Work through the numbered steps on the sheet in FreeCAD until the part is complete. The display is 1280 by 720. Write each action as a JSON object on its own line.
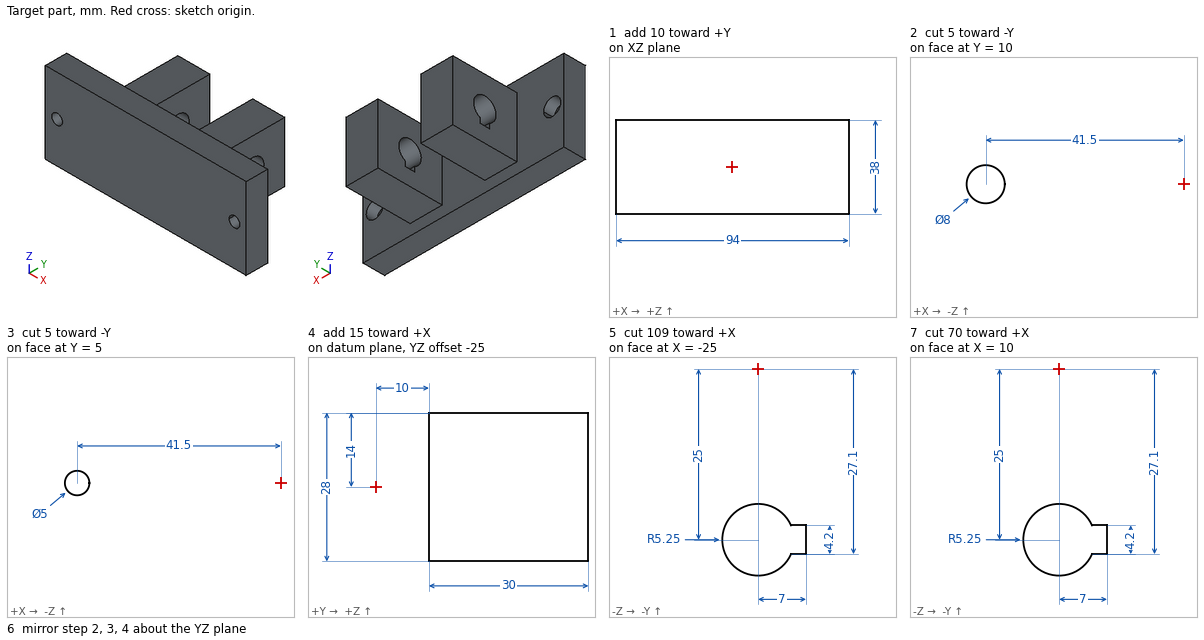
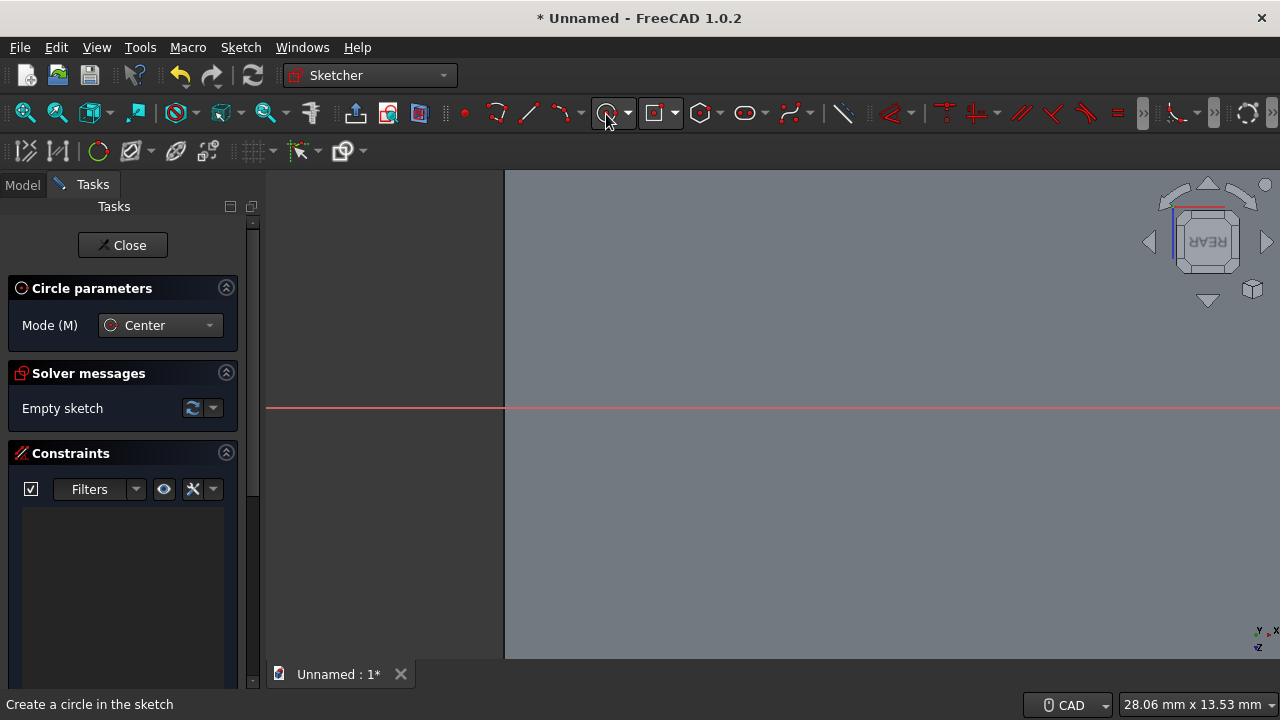
{"action": "left_click", "coordinate": [703, 408]}
{"action": "left_click", "coordinate": [805, 306]}
{"action": "key", "text": "Escape"}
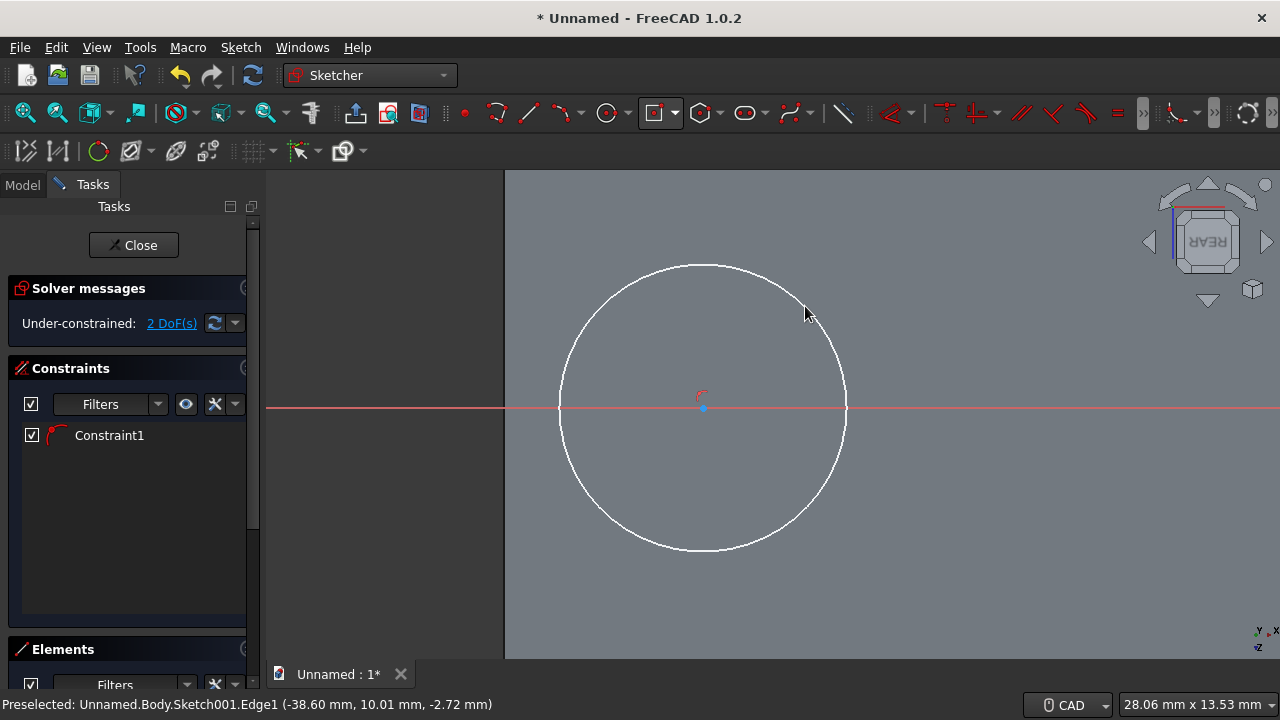
{"action": "left_click", "coordinate": [890, 114]}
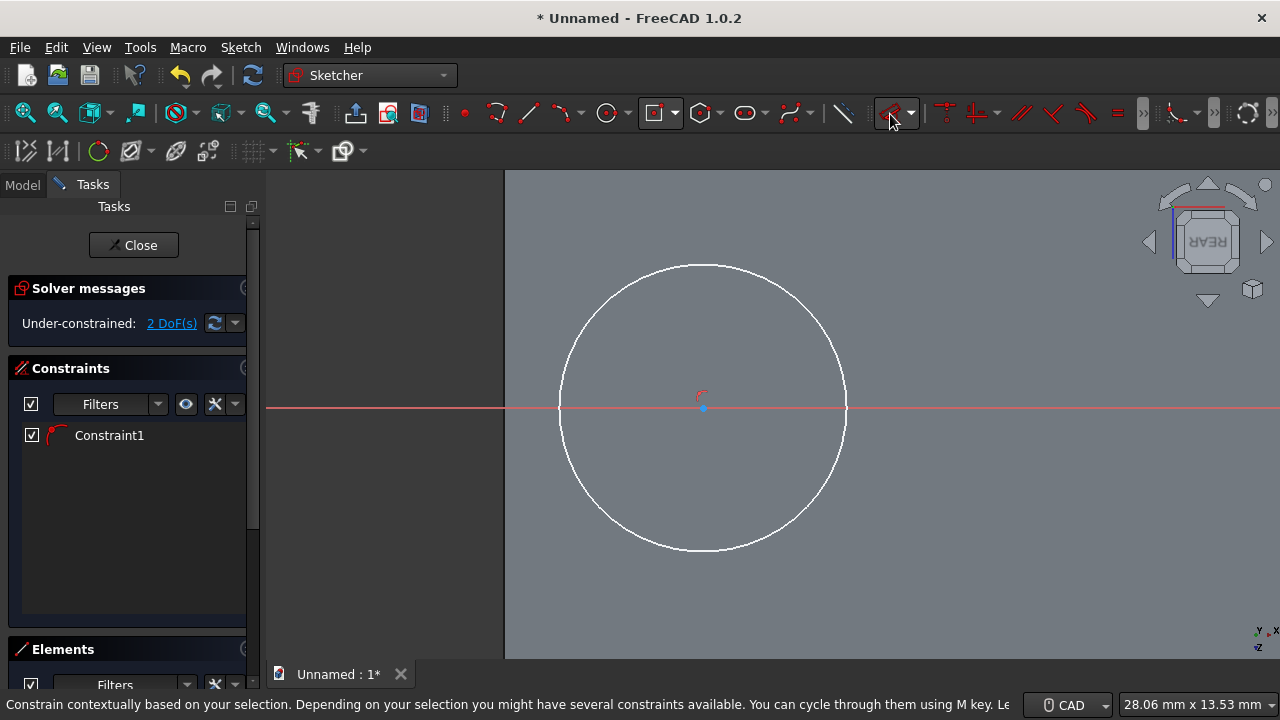
{"action": "left_click", "coordinate": [804, 306]}
{"action": "left_click", "coordinate": [827, 283]}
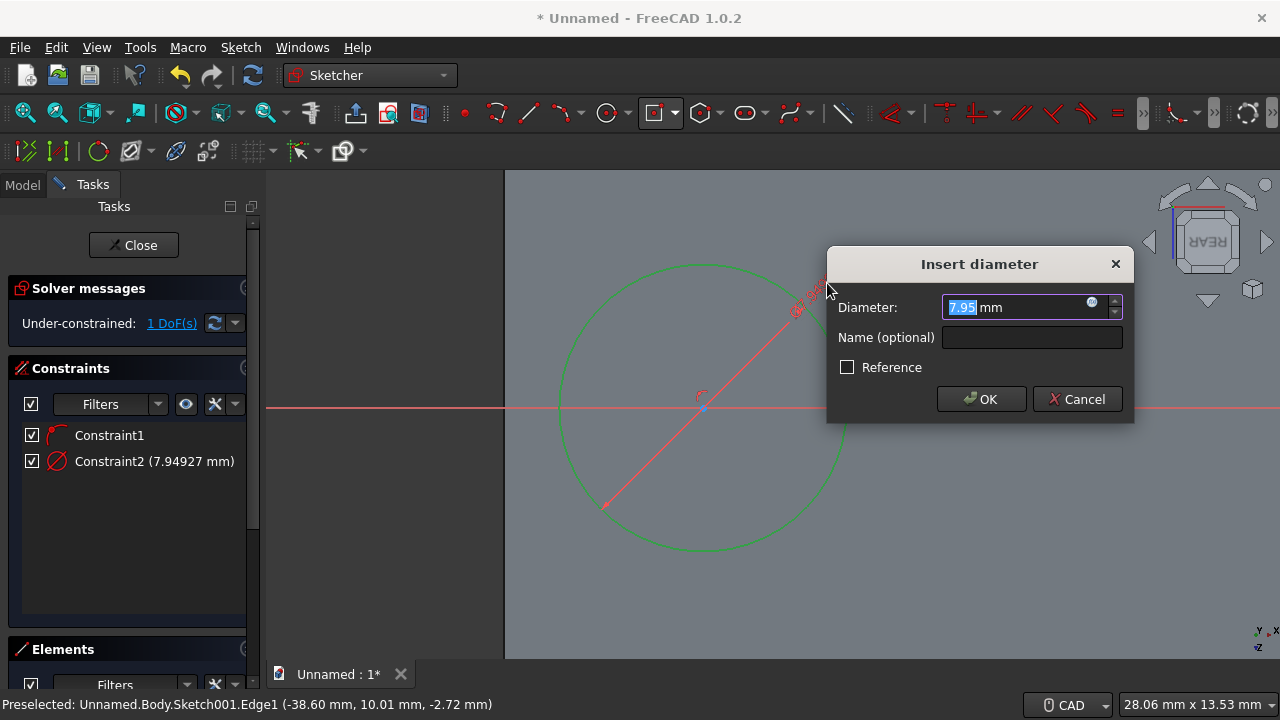
{"action": "type", "text": "8"}
{"action": "key", "text": "Return"}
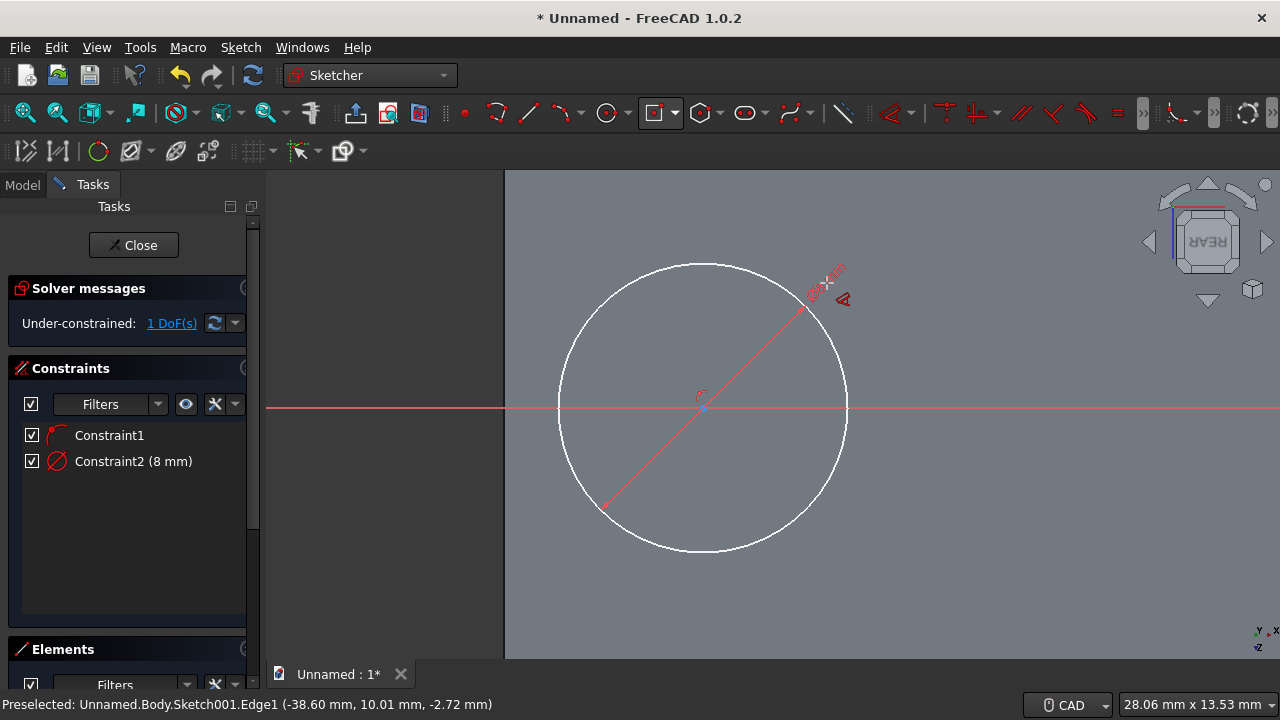
{"action": "left_click", "coordinate": [703, 408]}
{"action": "left_click", "coordinate": [909, 442]}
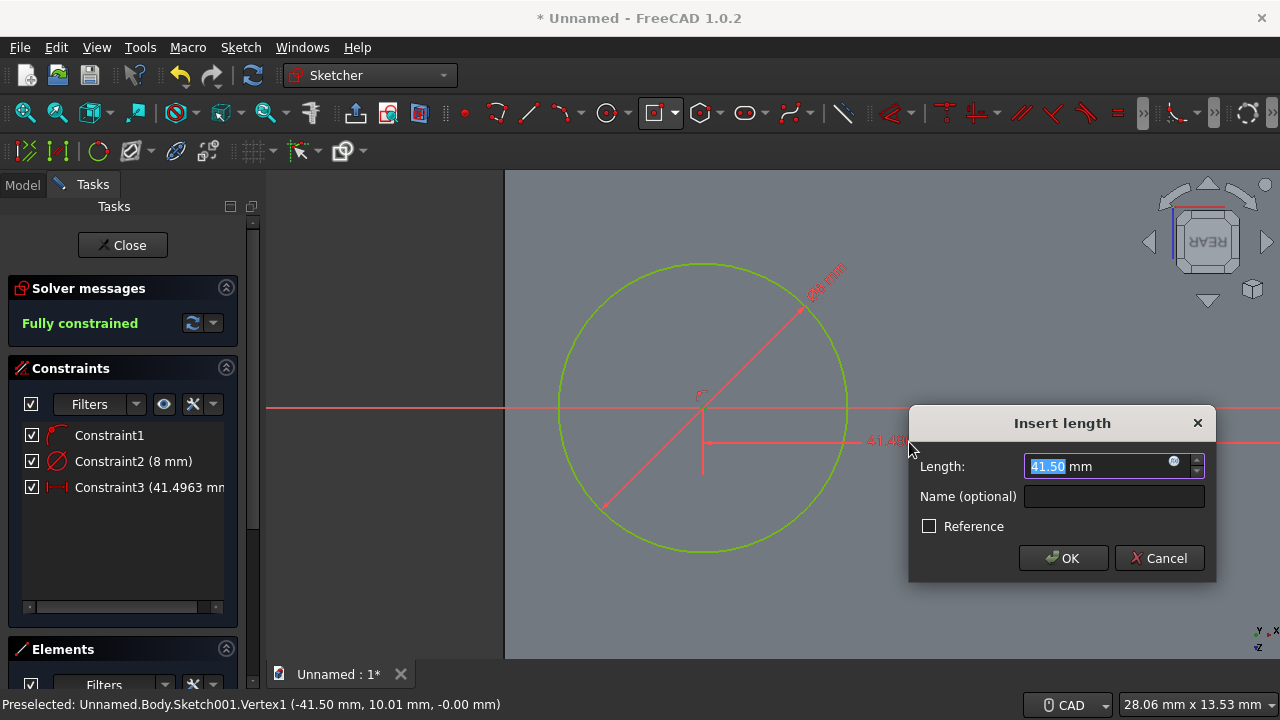
{"action": "type", "text": "41.5"}
{"action": "key", "text": "Return"}
{"action": "key", "text": "Escape"}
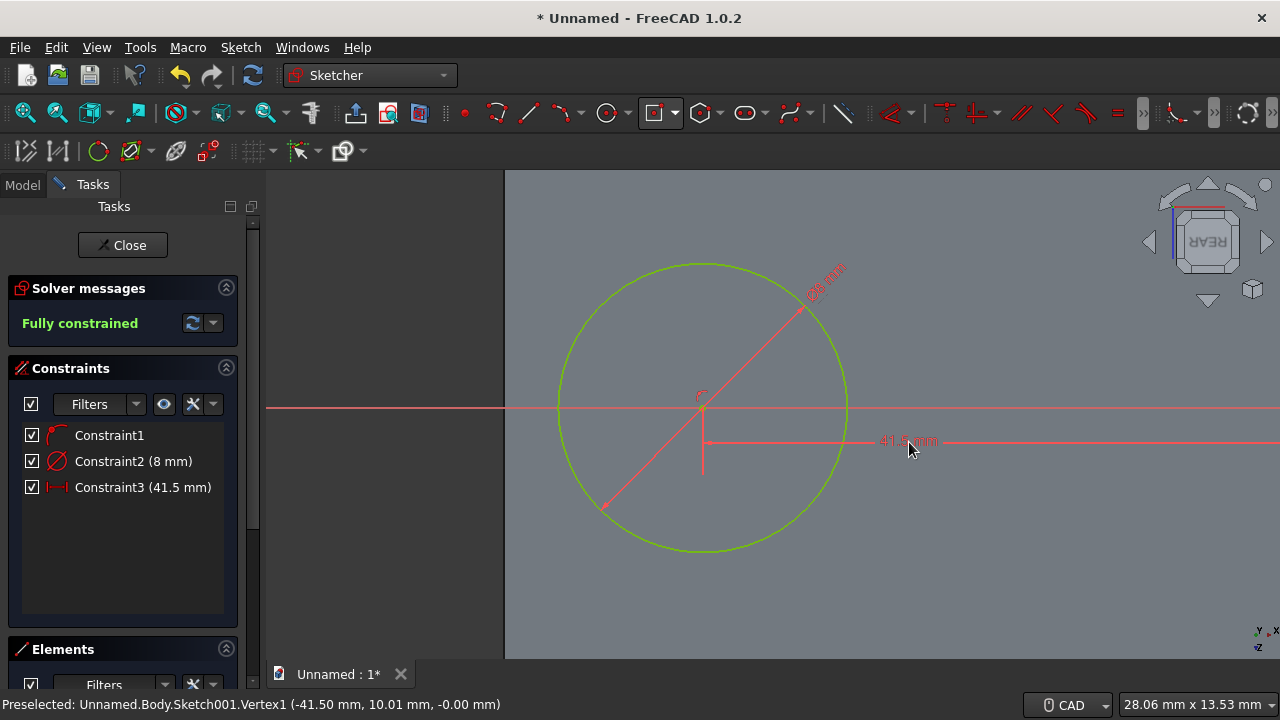
{"action": "left_click", "coordinate": [123, 245]}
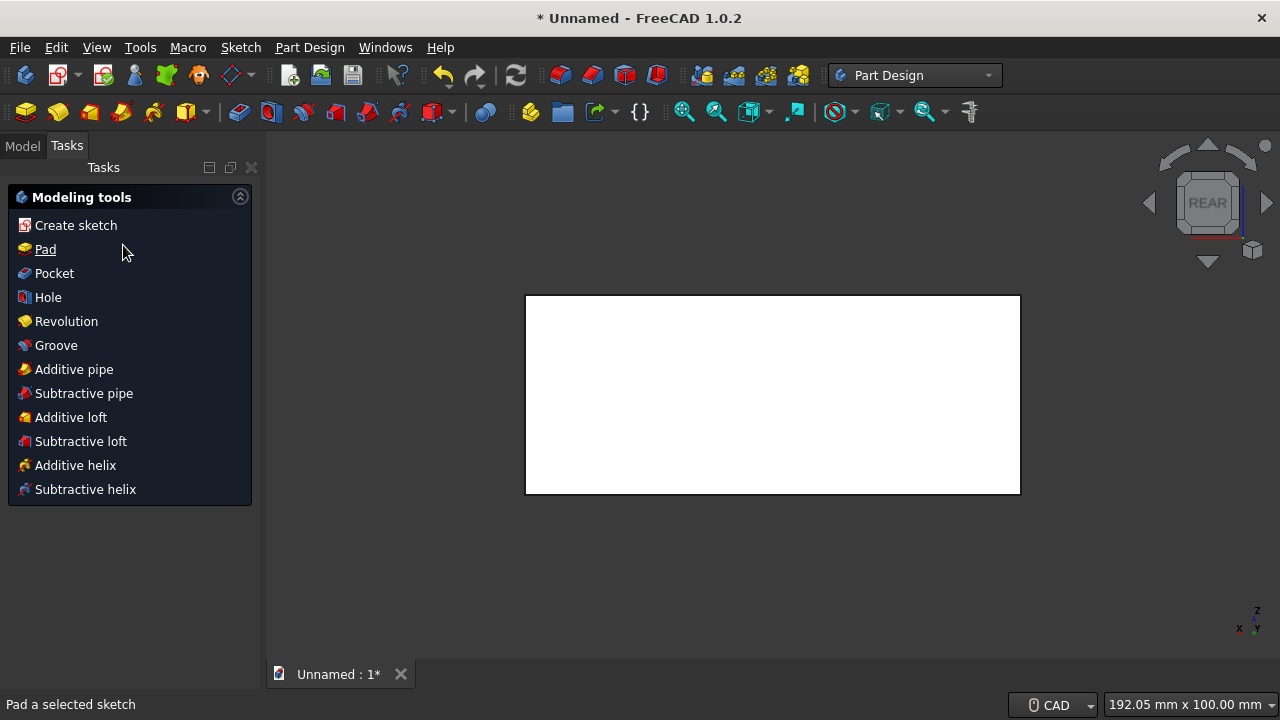
{"action": "left_click", "coordinate": [240, 112]}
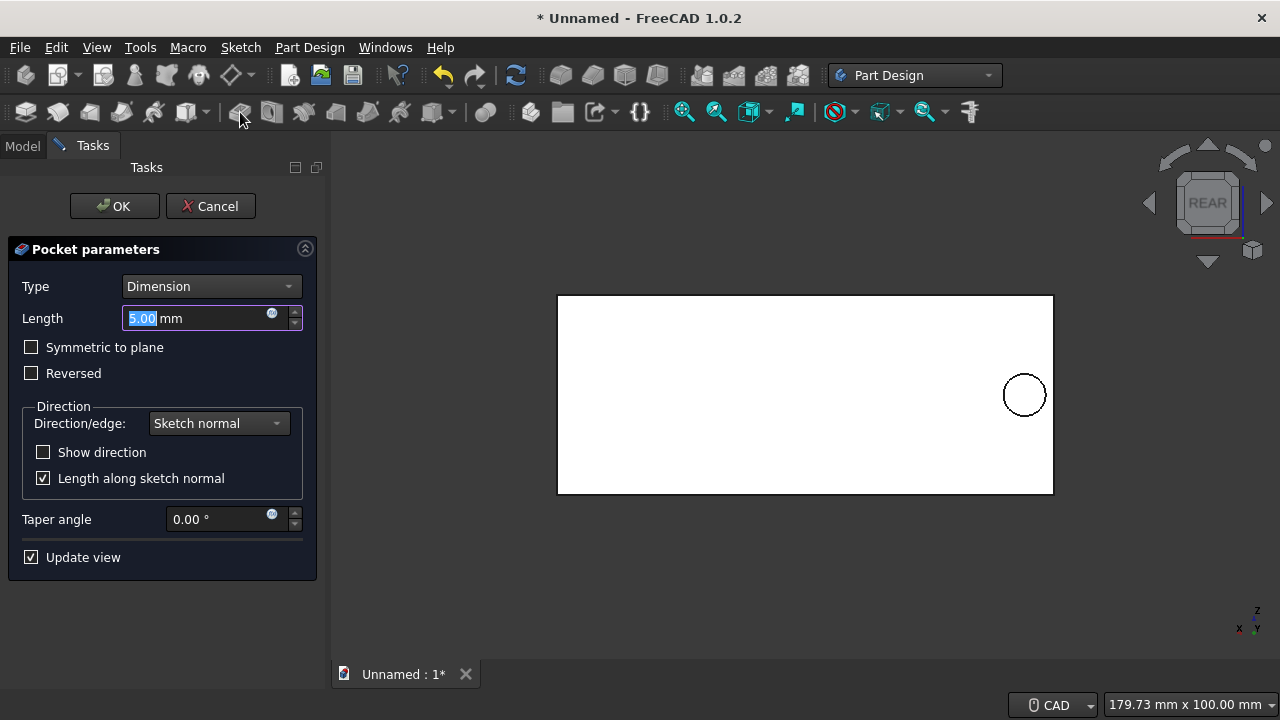
{"action": "type", "text": "5"}
{"action": "key", "text": "Tab"}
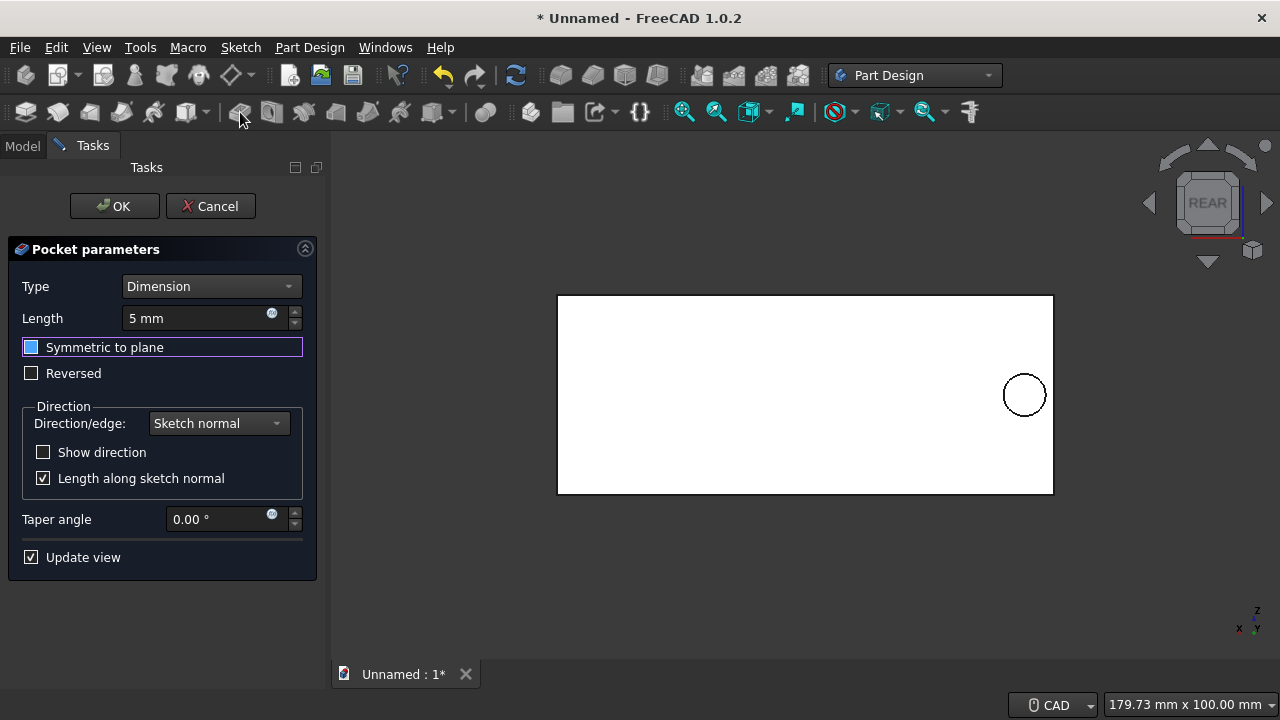
{"action": "left_click", "coordinate": [115, 206]}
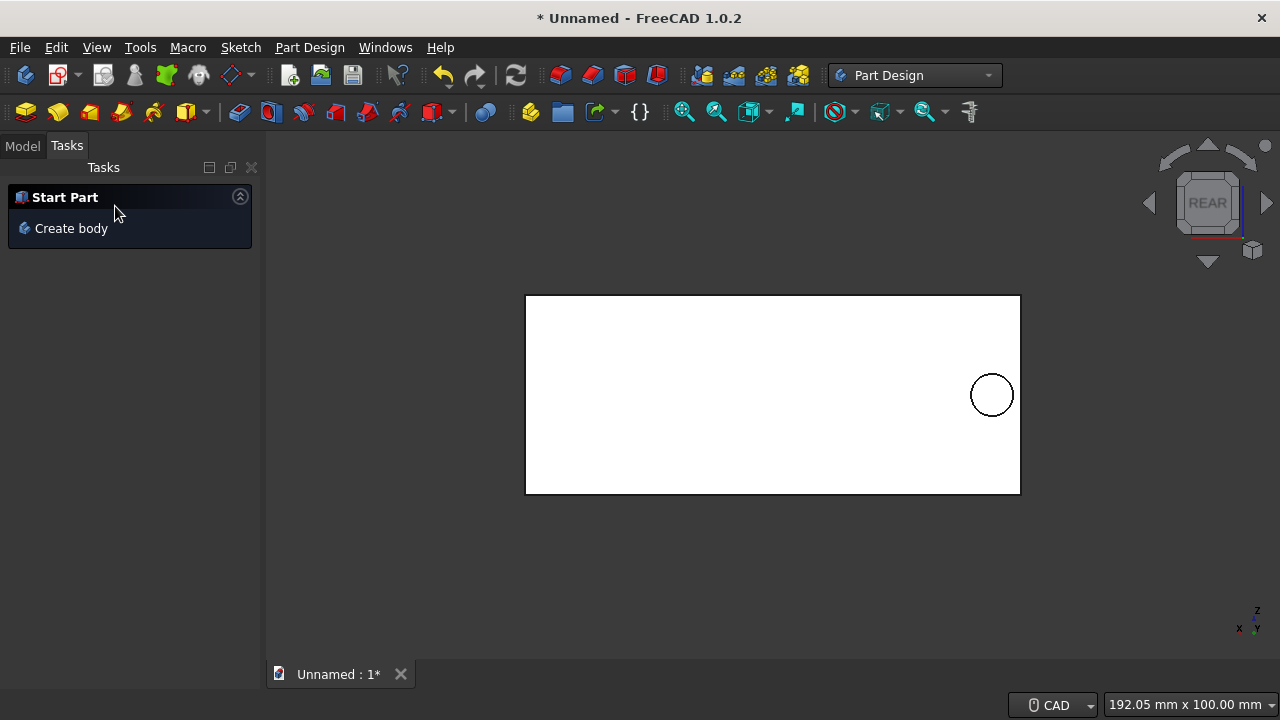
{"action": "left_click", "coordinate": [992, 394]}